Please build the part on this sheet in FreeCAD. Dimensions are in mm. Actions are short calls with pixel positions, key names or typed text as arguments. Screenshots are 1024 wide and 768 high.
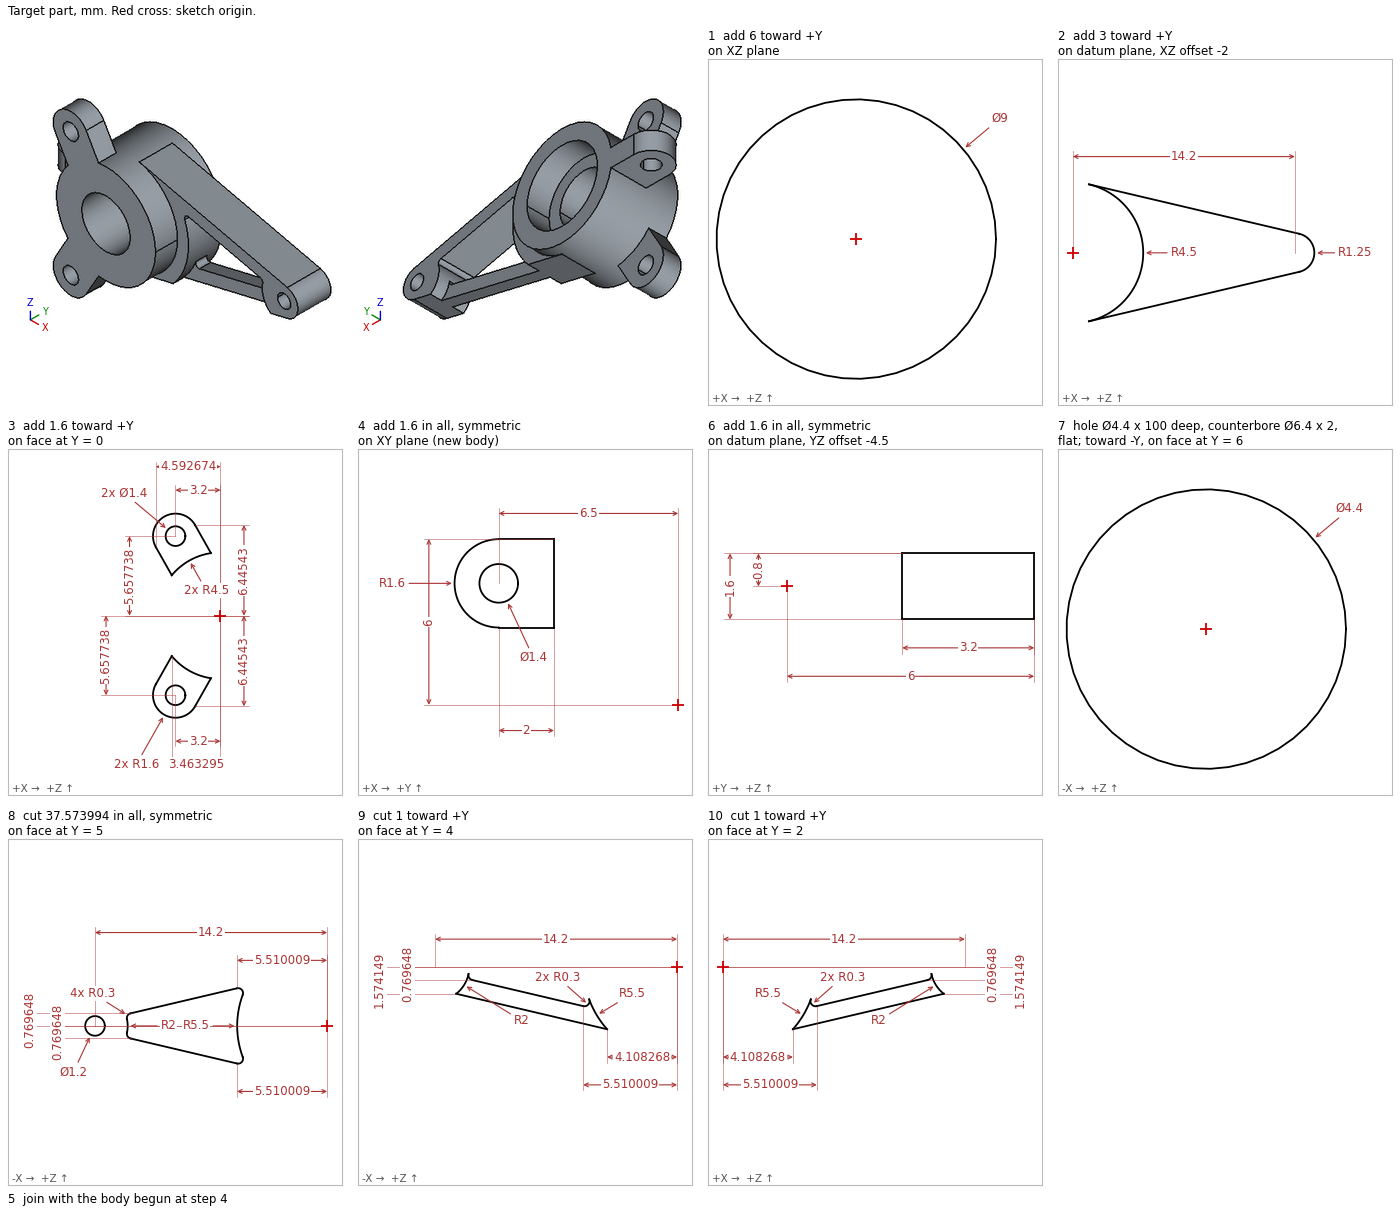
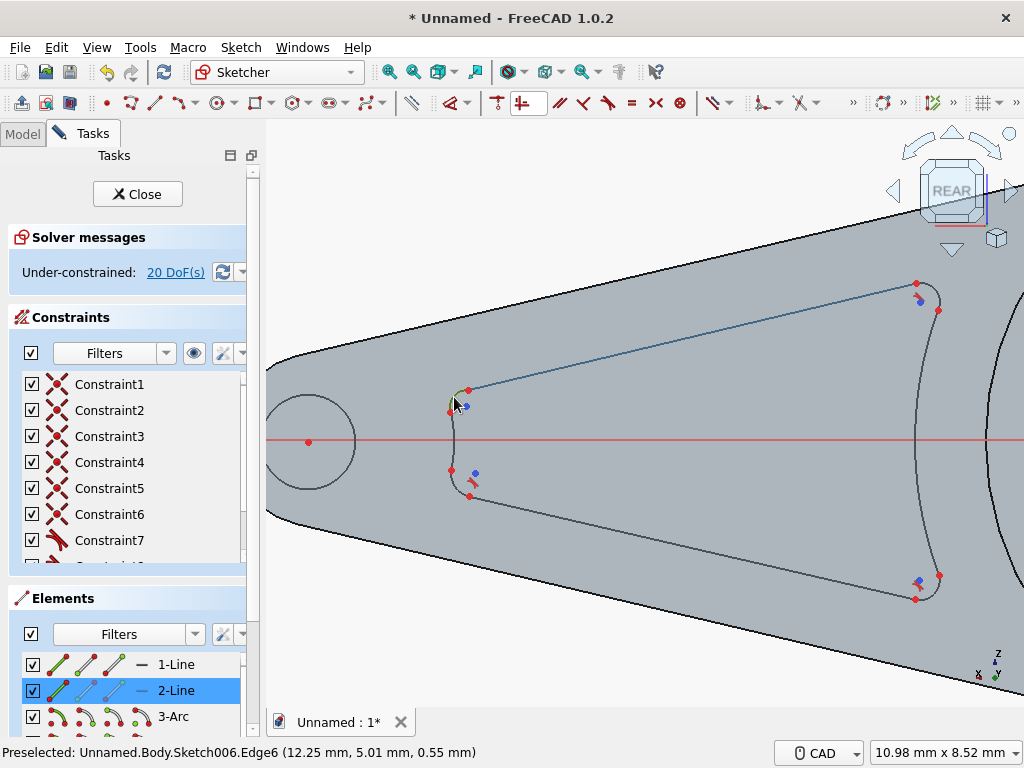
key(t)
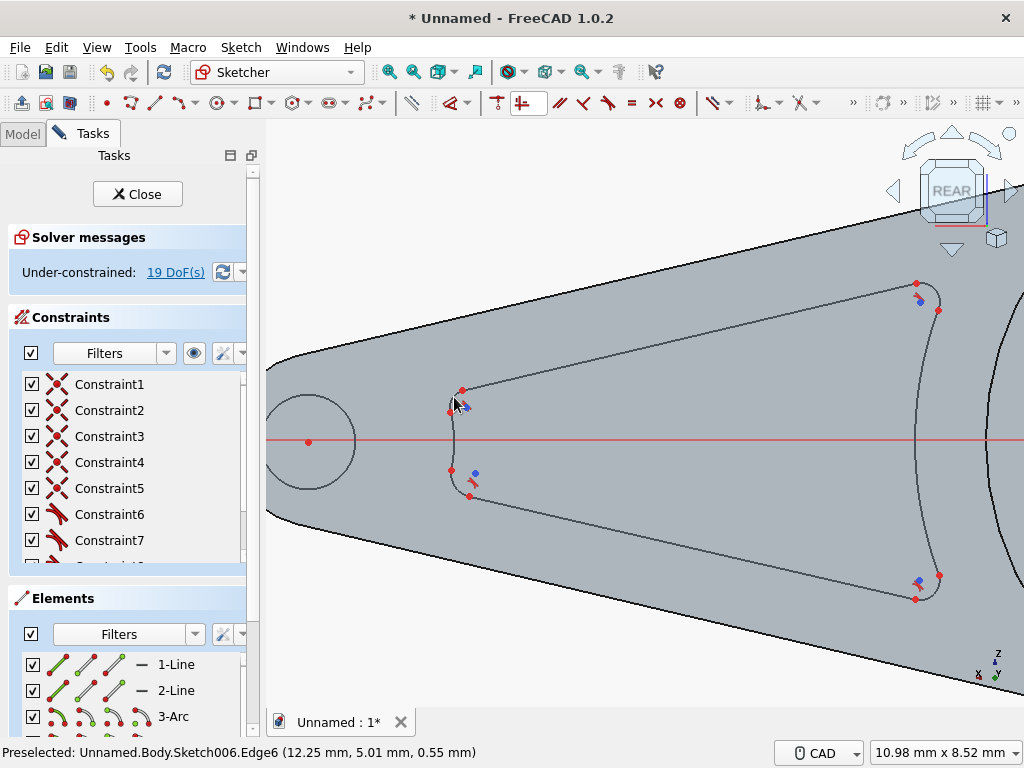
scroll(455, 397, down, 5)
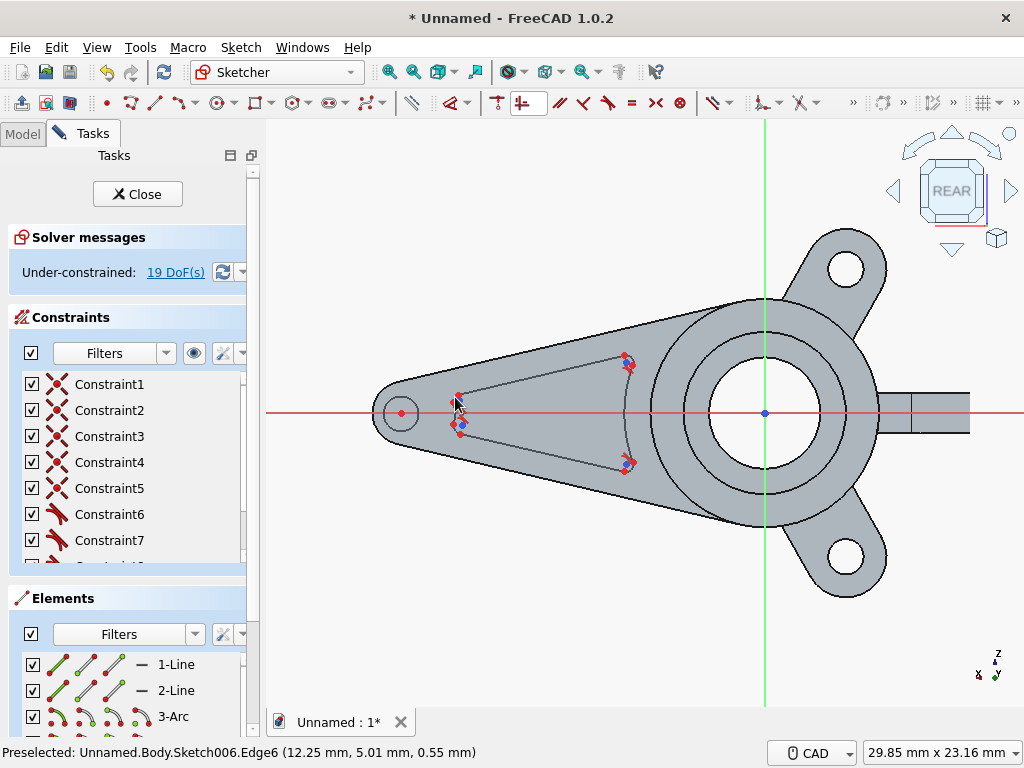
scroll(629, 471, up, 6)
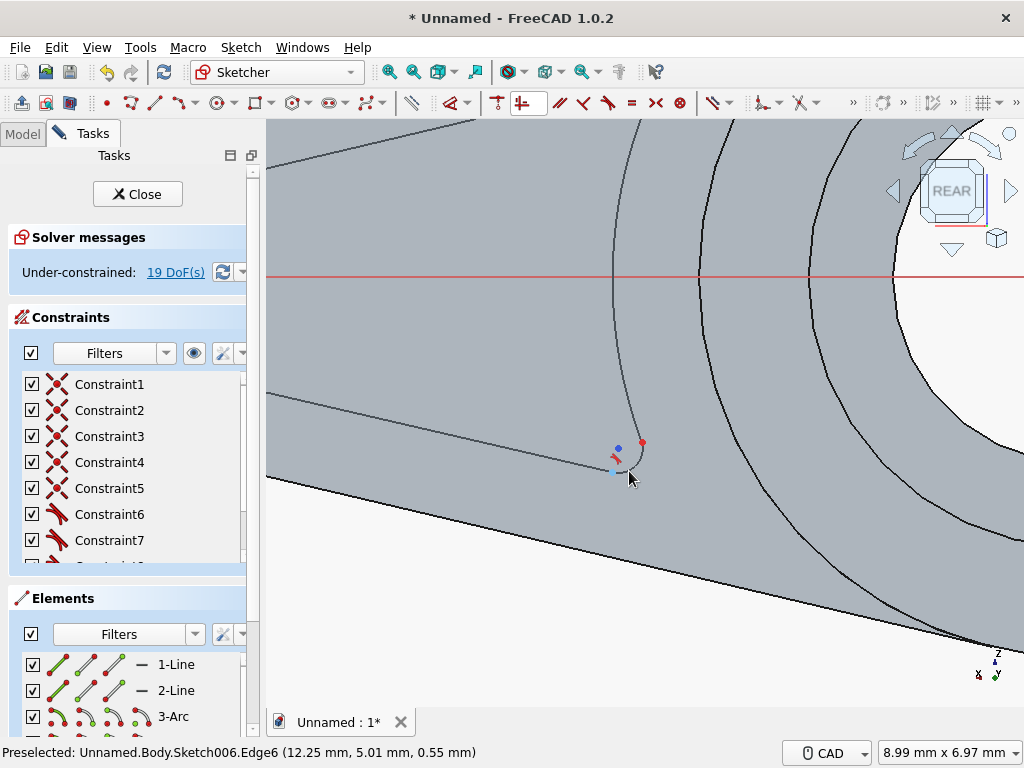
click(627, 471)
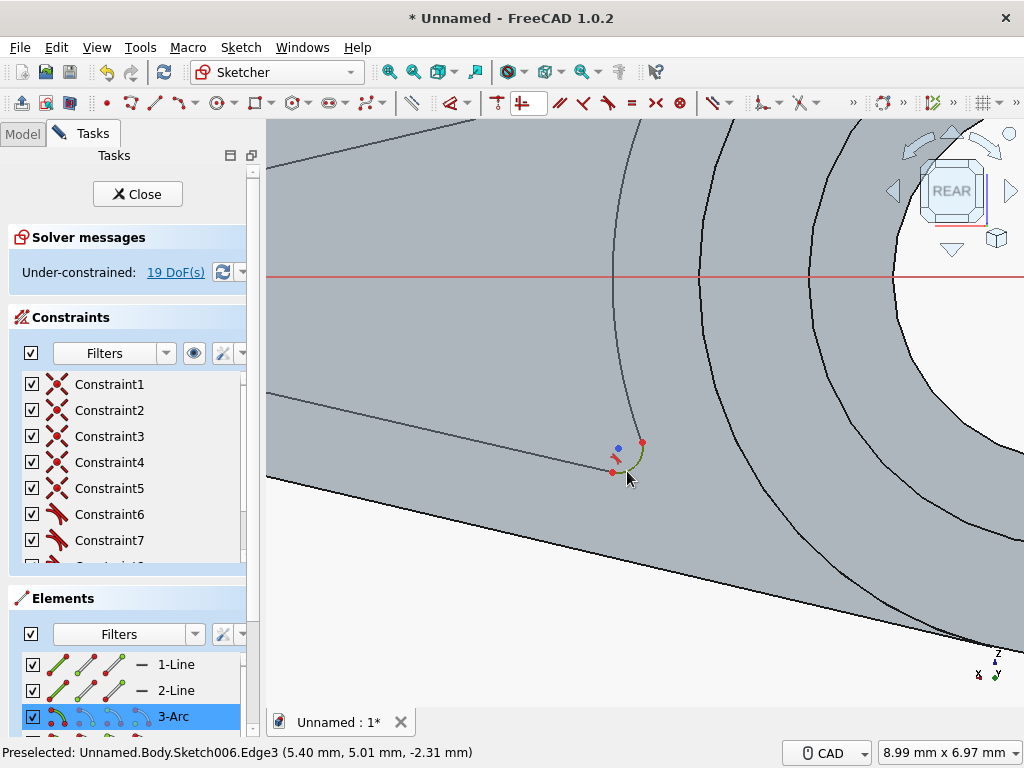
scroll(629, 471, down, 6)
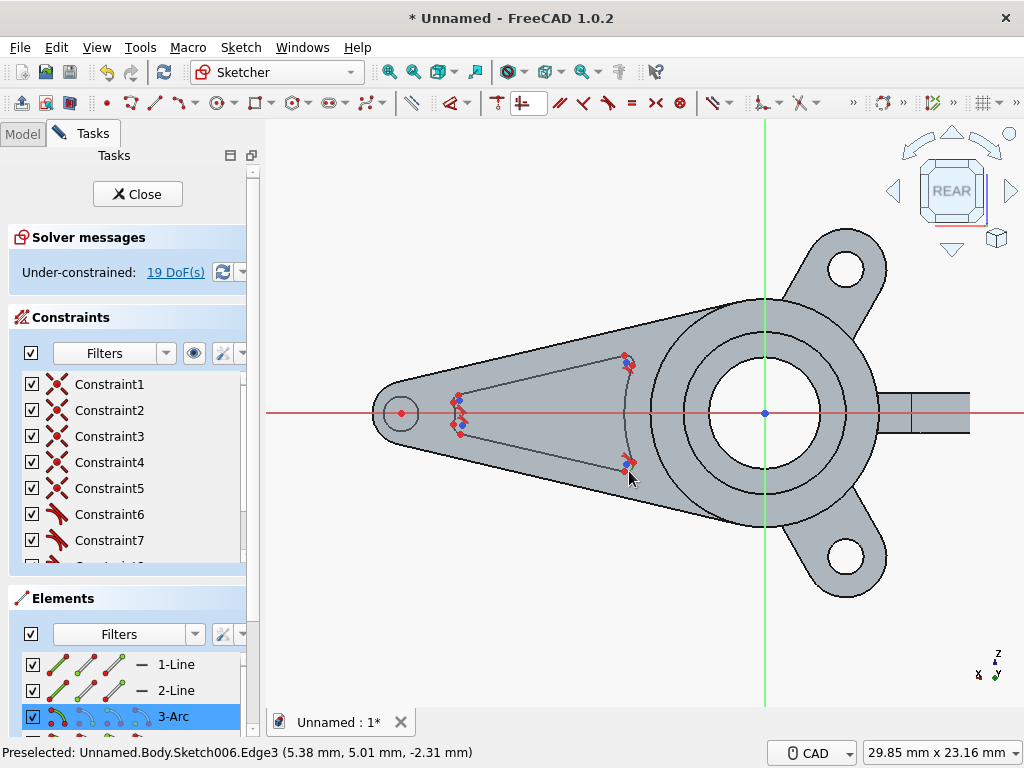
click(626, 394)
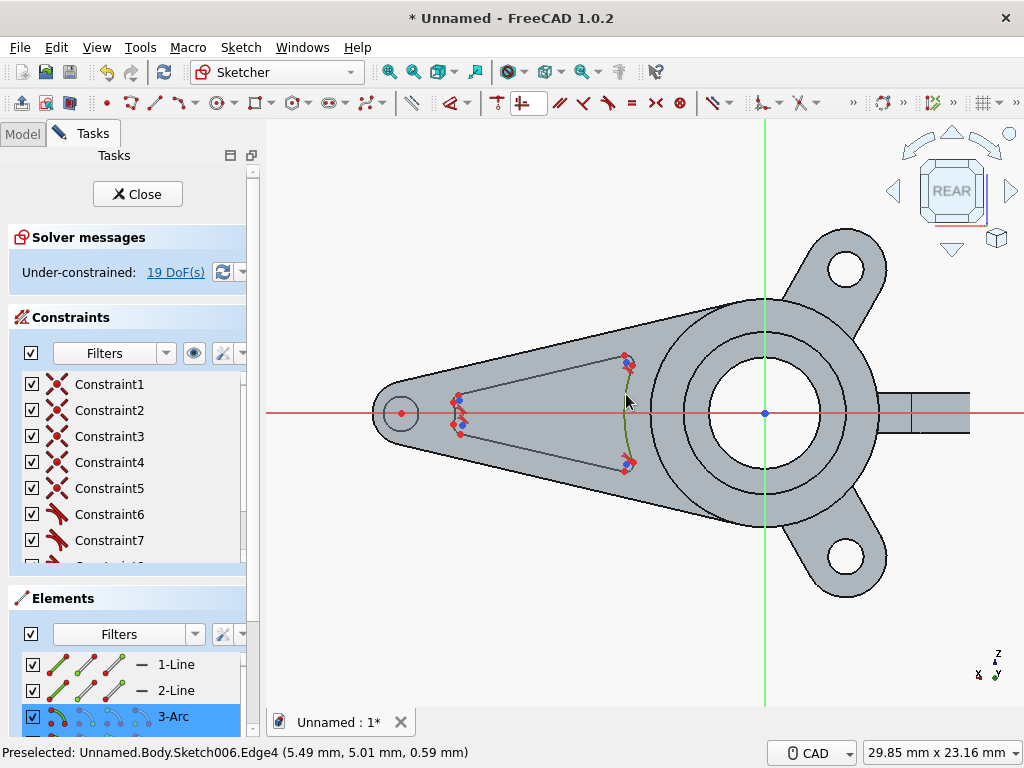
key(t)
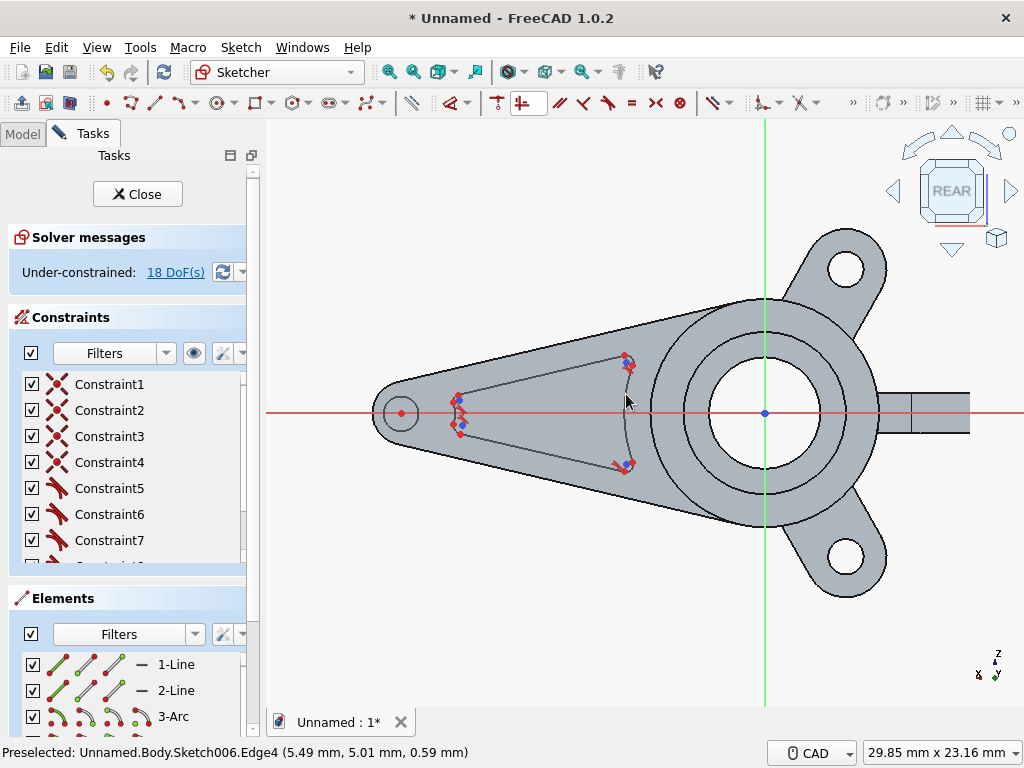
click(626, 394)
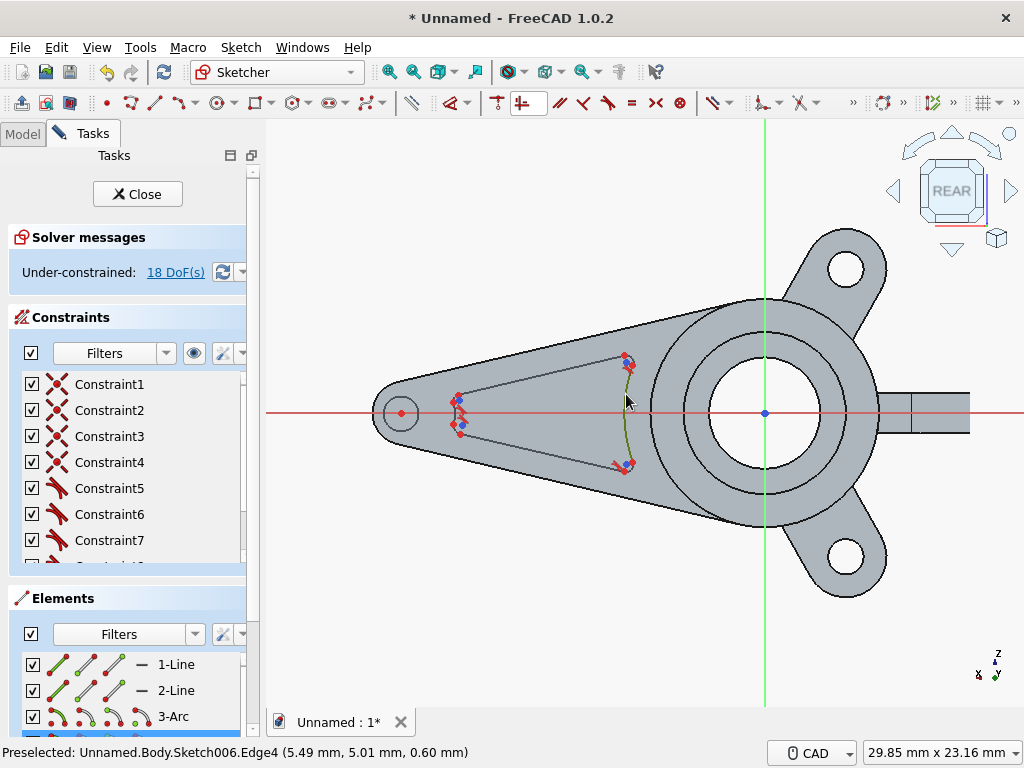
scroll(632, 358, up, 4)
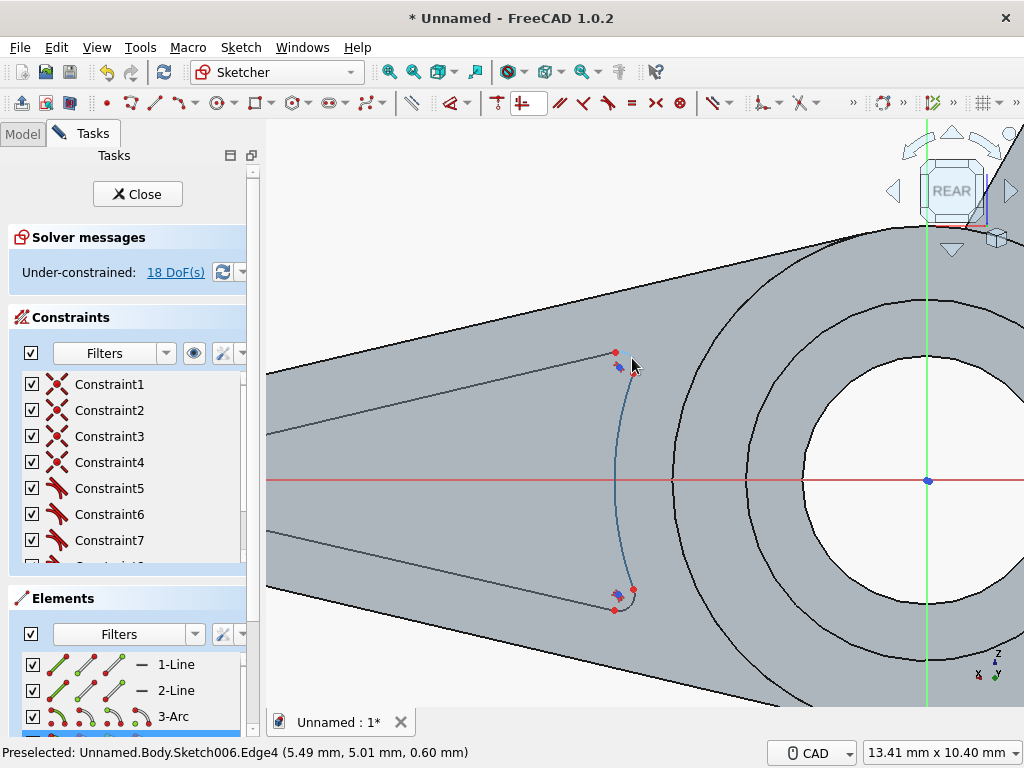
click(631, 357)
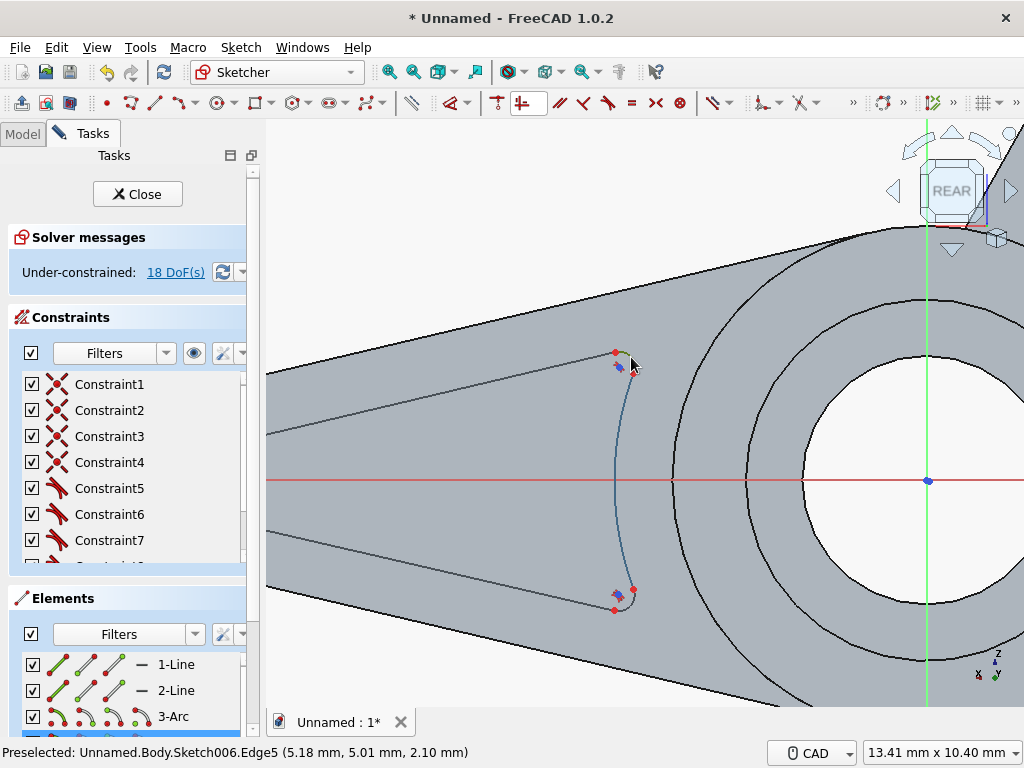
key(t)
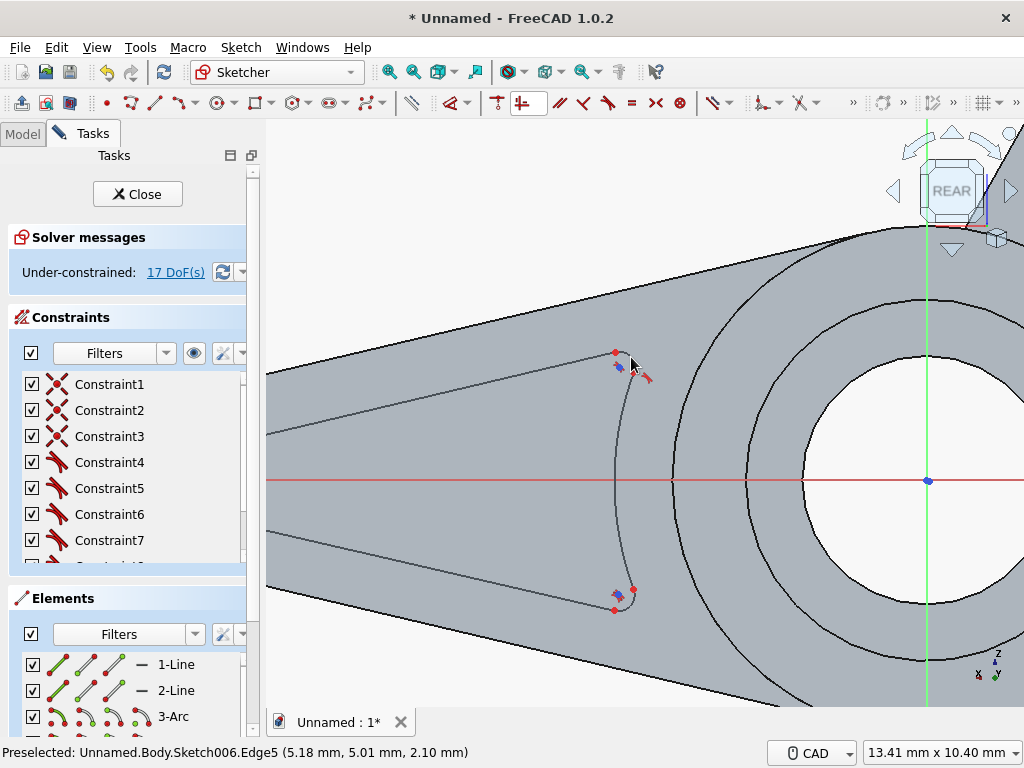
scroll(632, 358, down, 4)